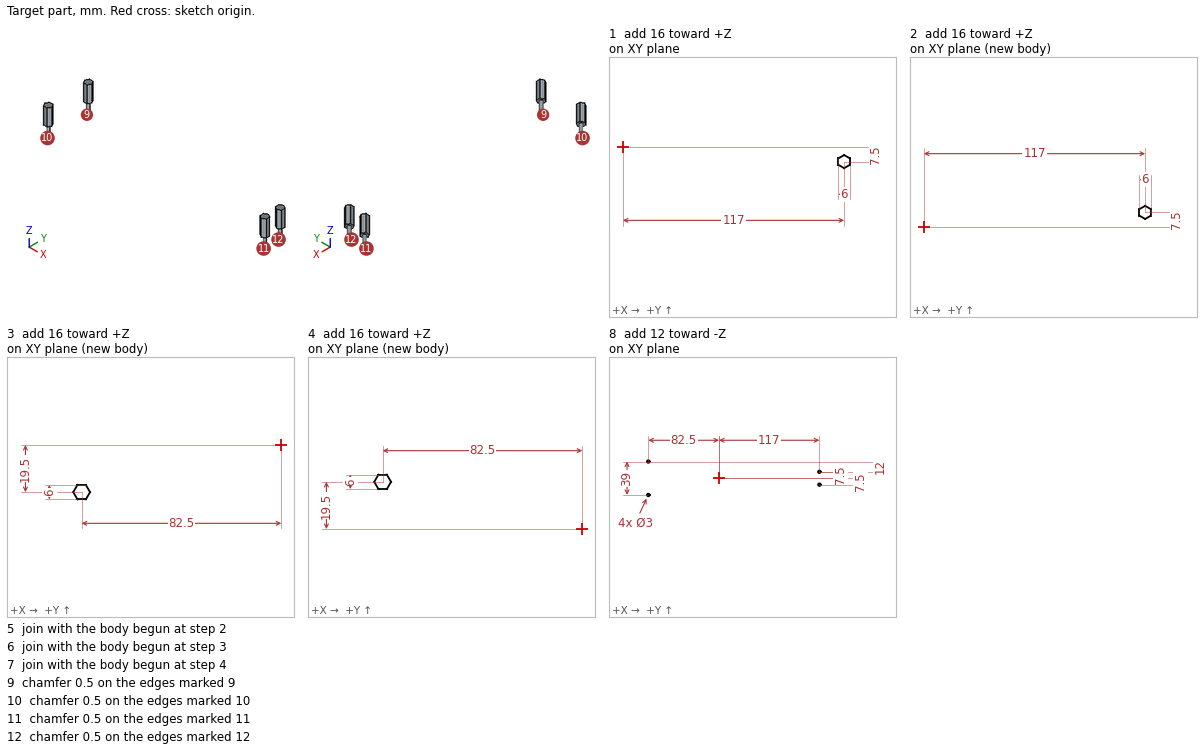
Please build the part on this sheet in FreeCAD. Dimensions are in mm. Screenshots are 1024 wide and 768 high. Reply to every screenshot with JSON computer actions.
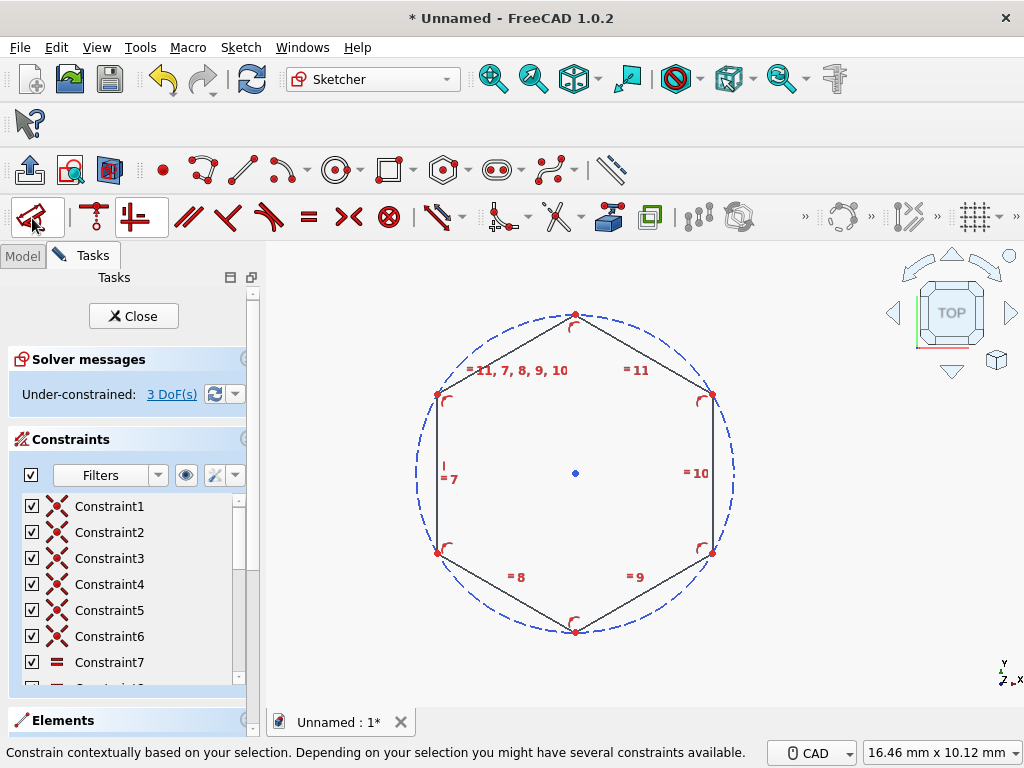
{"action": "left_click", "coordinate": [437, 395]}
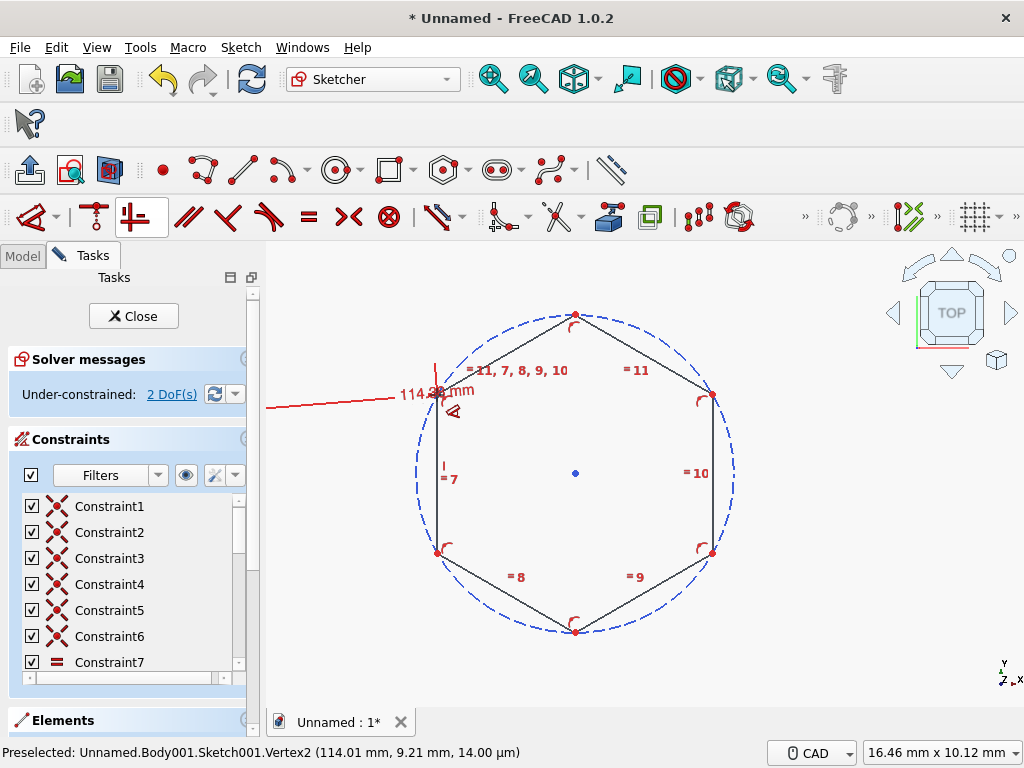
{"action": "left_click", "coordinate": [713, 554]}
{"action": "left_click", "coordinate": [575, 588]}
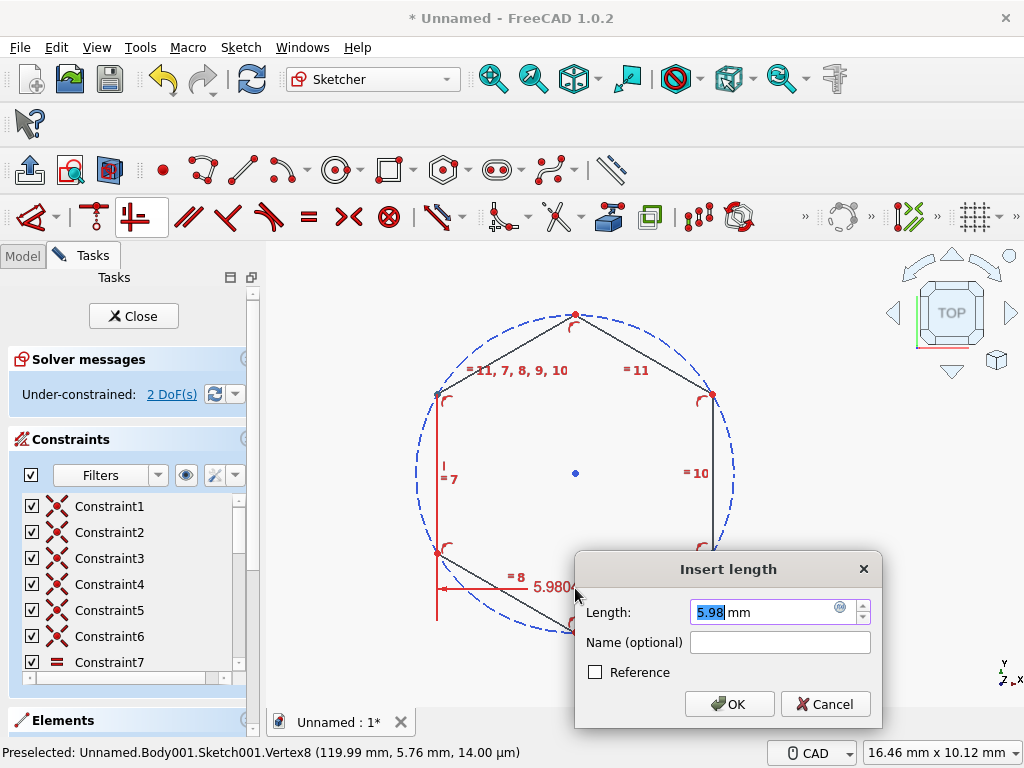
{"action": "type", "text": "6"}
{"action": "key", "text": "Return"}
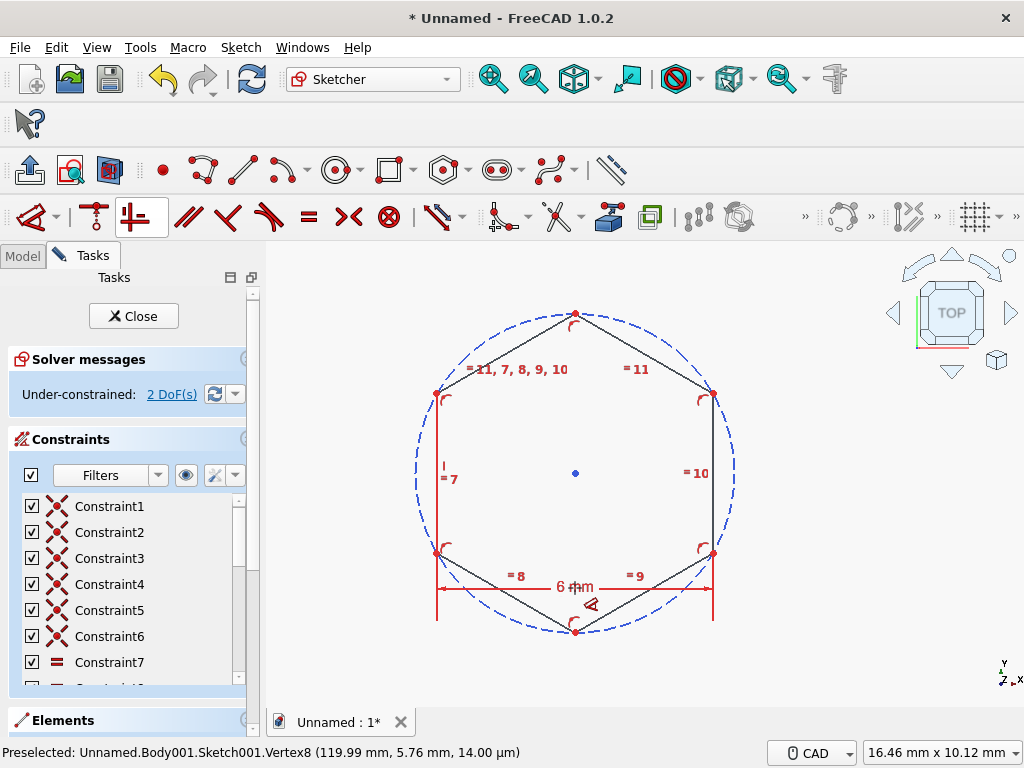
{"action": "left_click", "coordinate": [575, 473]}
{"action": "left_click", "coordinate": [370, 439]}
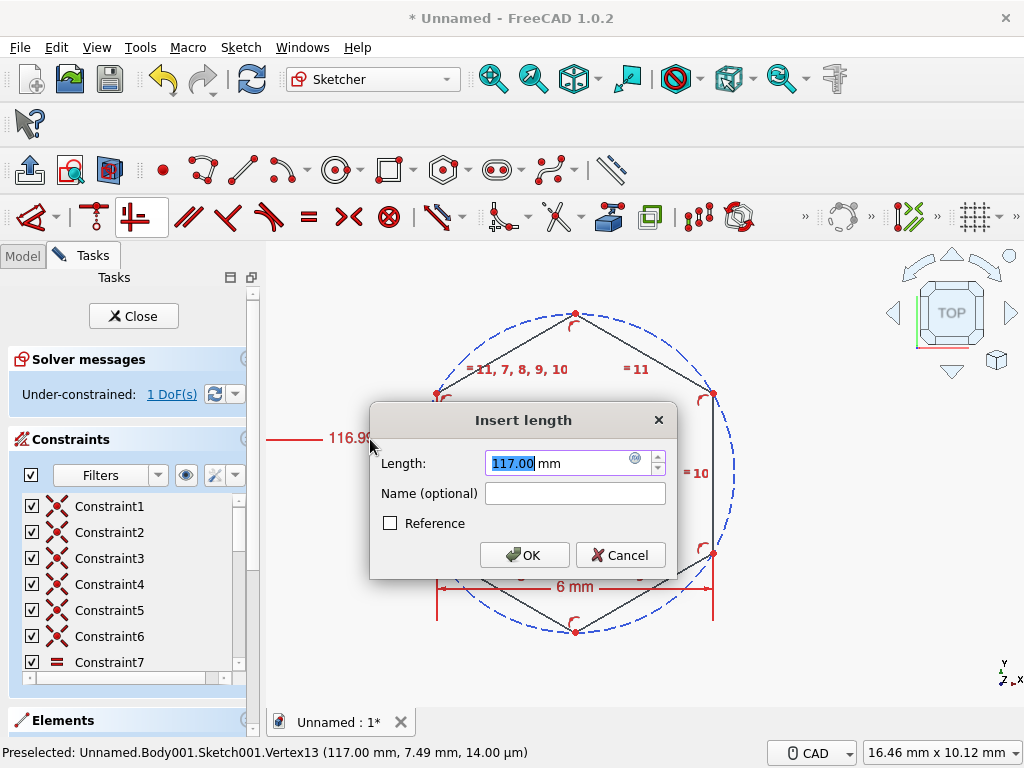
{"action": "type", "text": "117"}
{"action": "key", "text": "Return"}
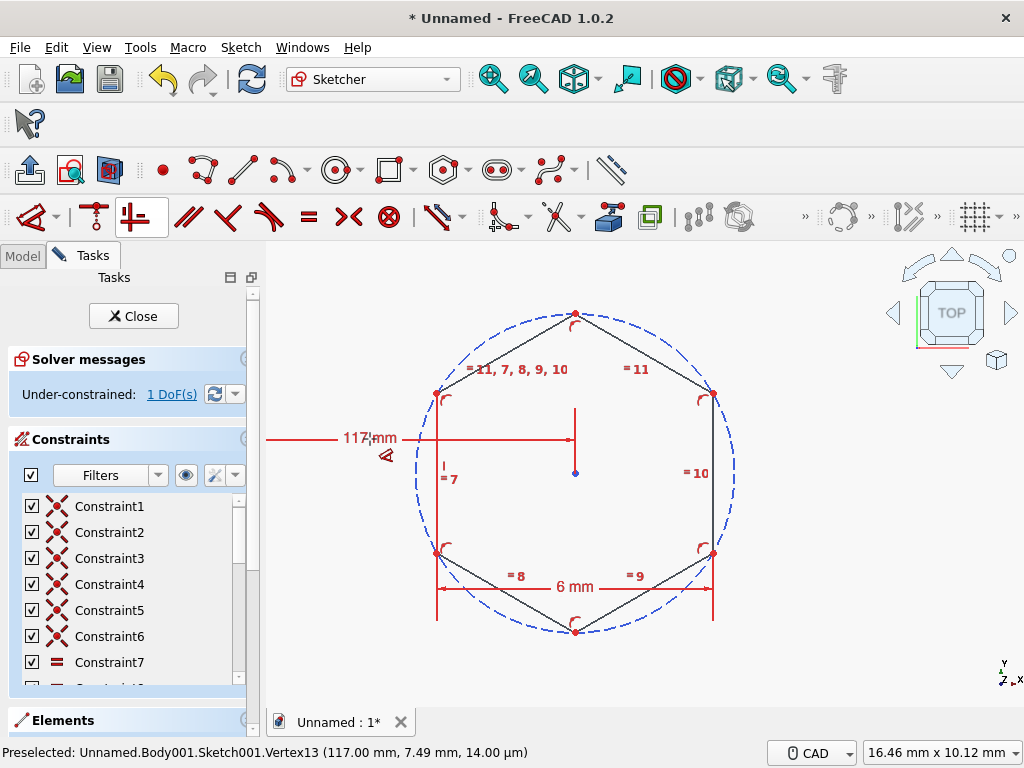
{"action": "left_click", "coordinate": [575, 473]}
{"action": "left_click", "coordinate": [609, 529]}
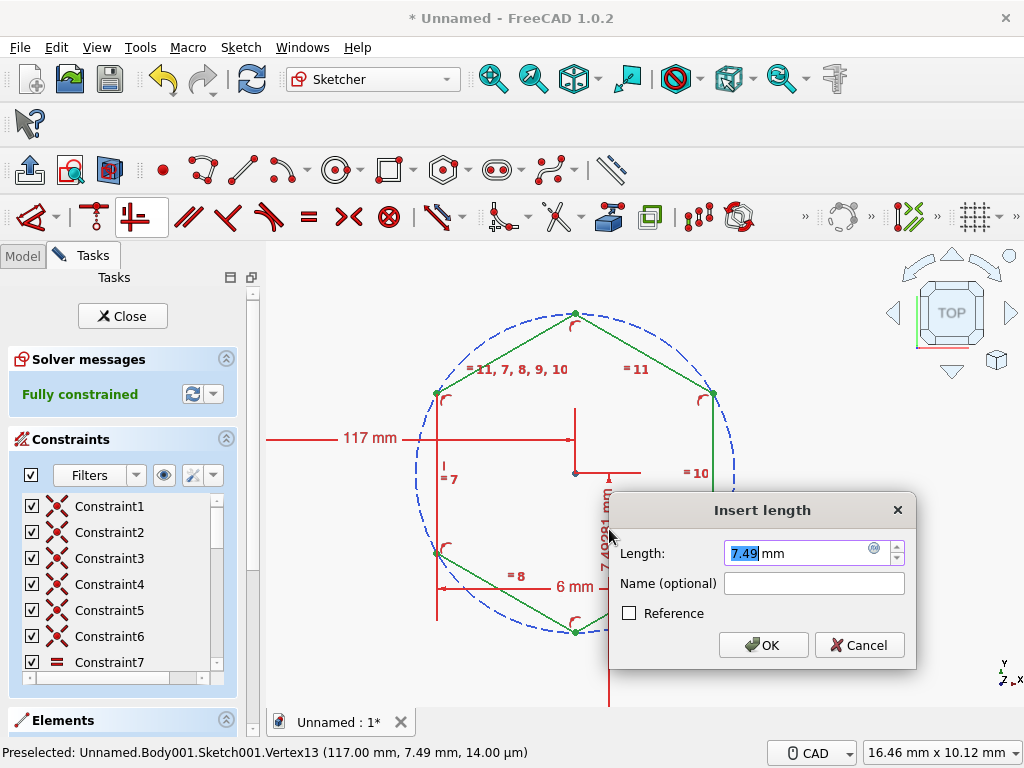
{"action": "type", "text": "7.5"}
{"action": "key", "text": "Return"}
{"action": "key", "text": "Escape"}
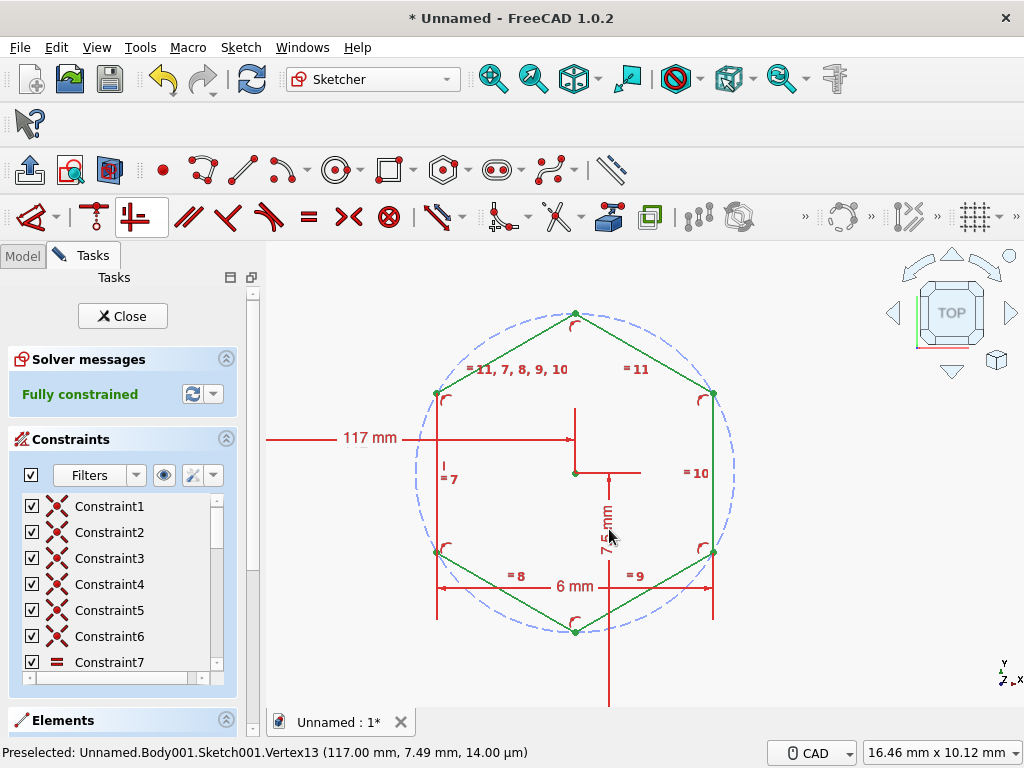
{"action": "left_click", "coordinate": [123, 316]}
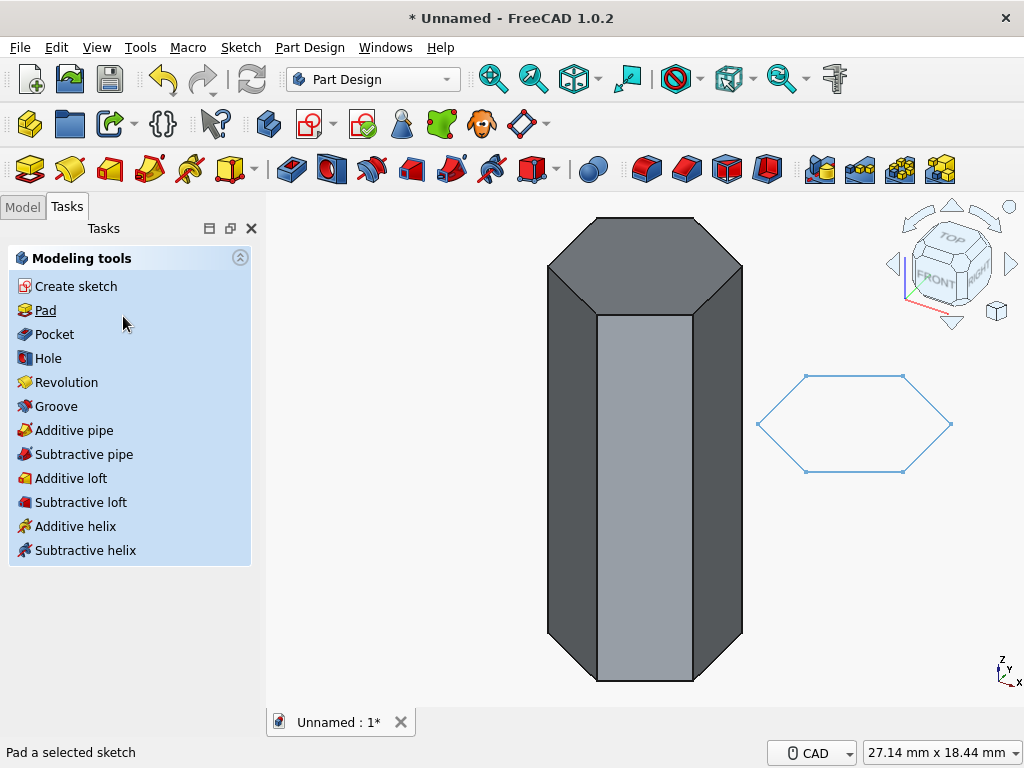
{"action": "left_click", "coordinate": [30, 170]}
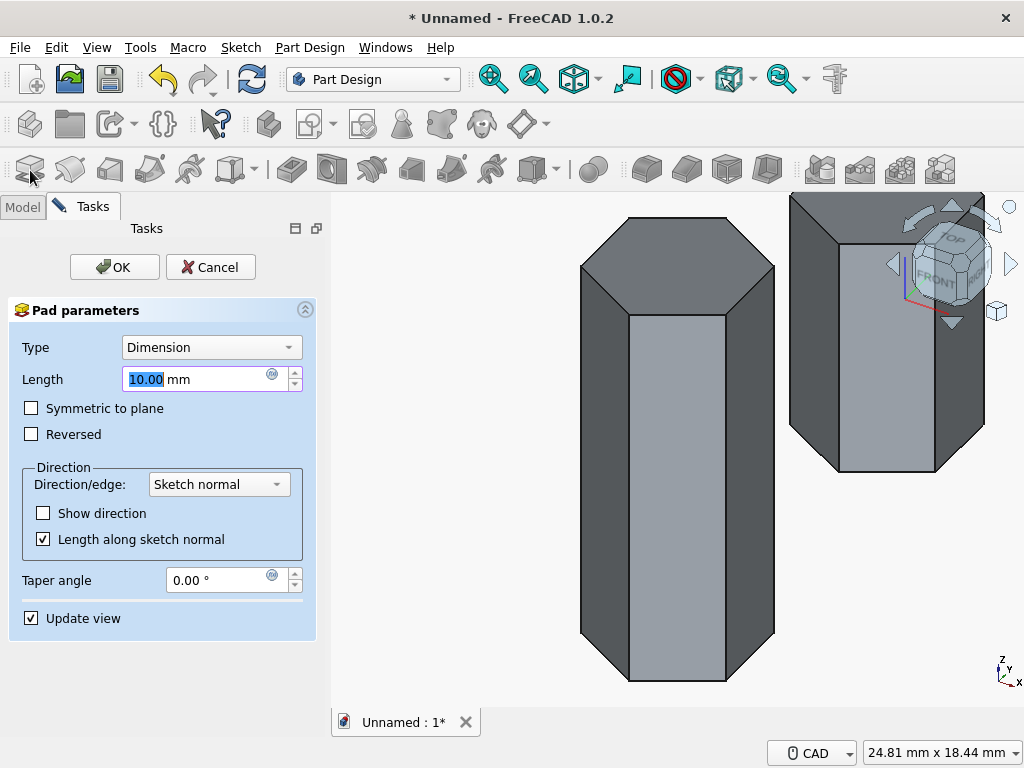
{"action": "type", "text": "16"}
{"action": "key", "text": "Tab"}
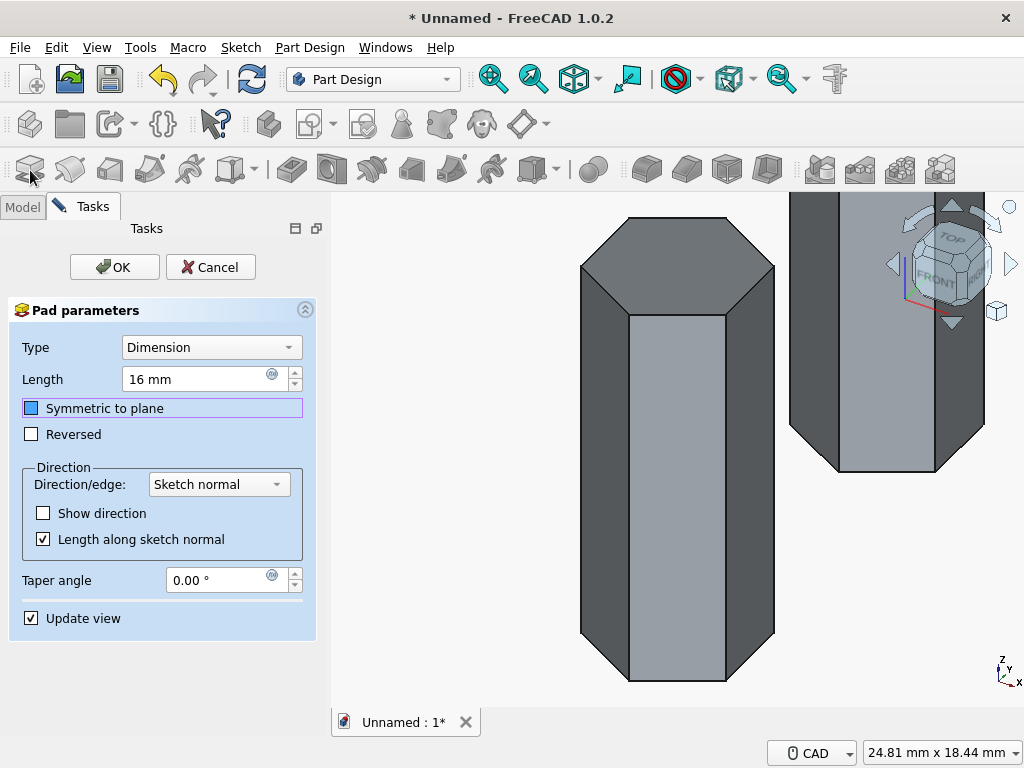
{"action": "left_click", "coordinate": [115, 267]}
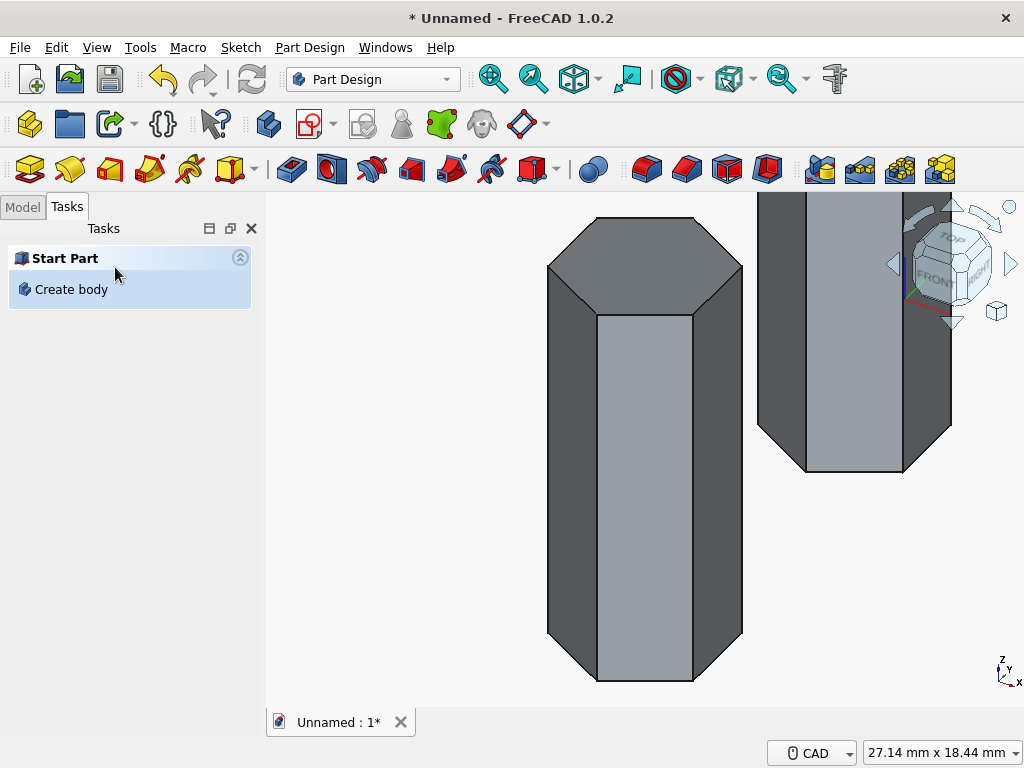
{"action": "left_click", "coordinate": [494, 80]}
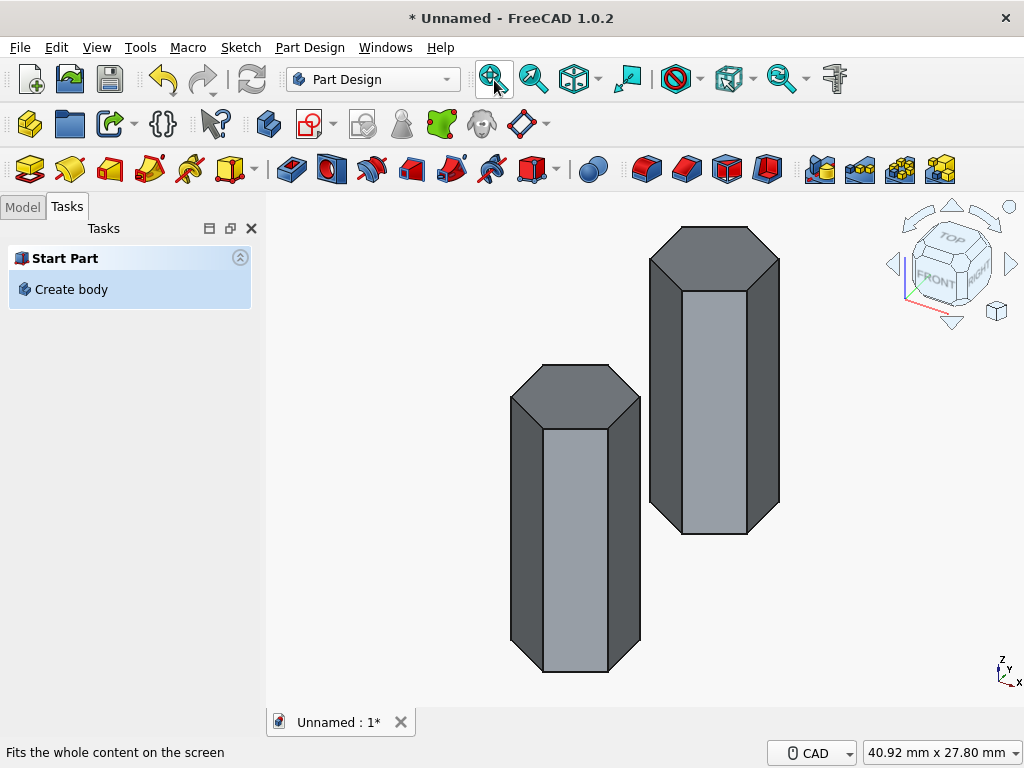
{"action": "left_click", "coordinate": [270, 124]}